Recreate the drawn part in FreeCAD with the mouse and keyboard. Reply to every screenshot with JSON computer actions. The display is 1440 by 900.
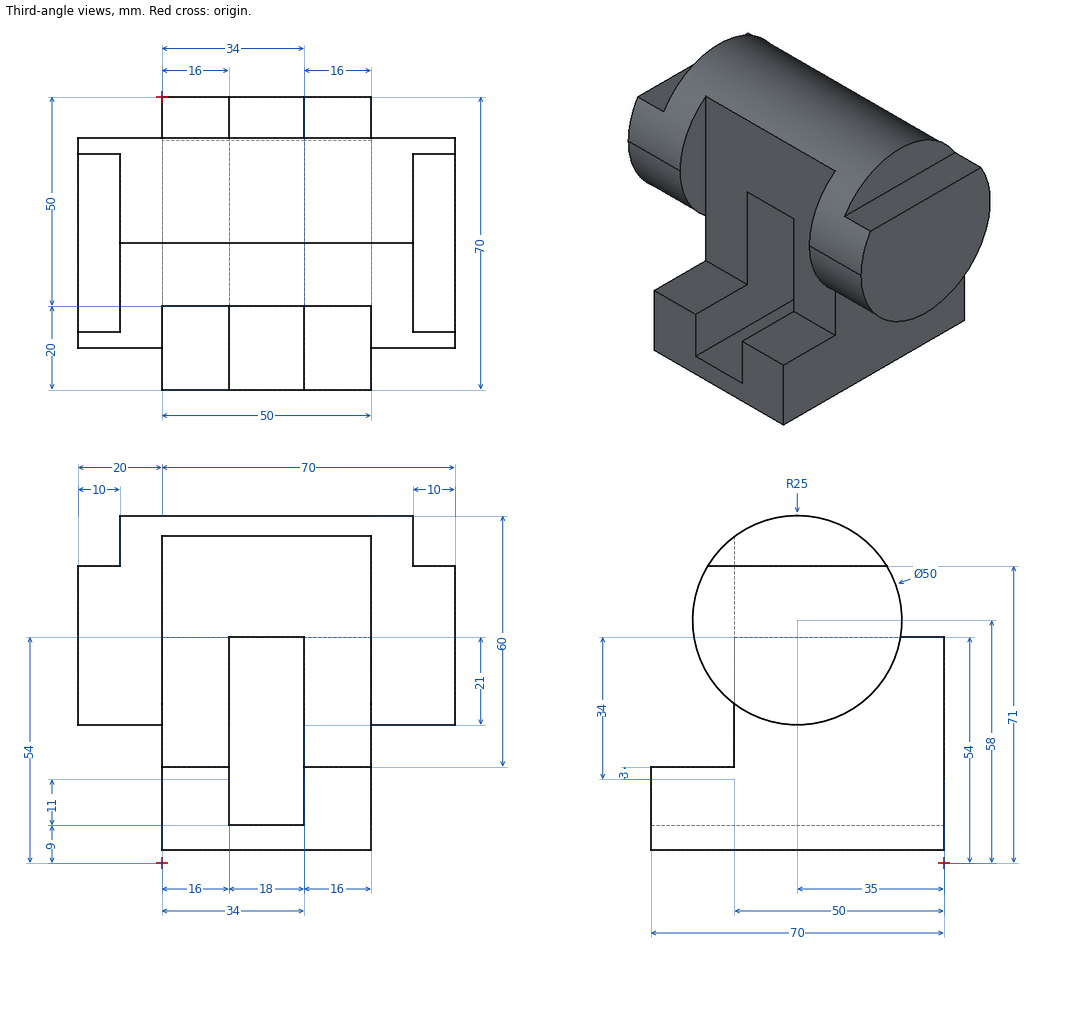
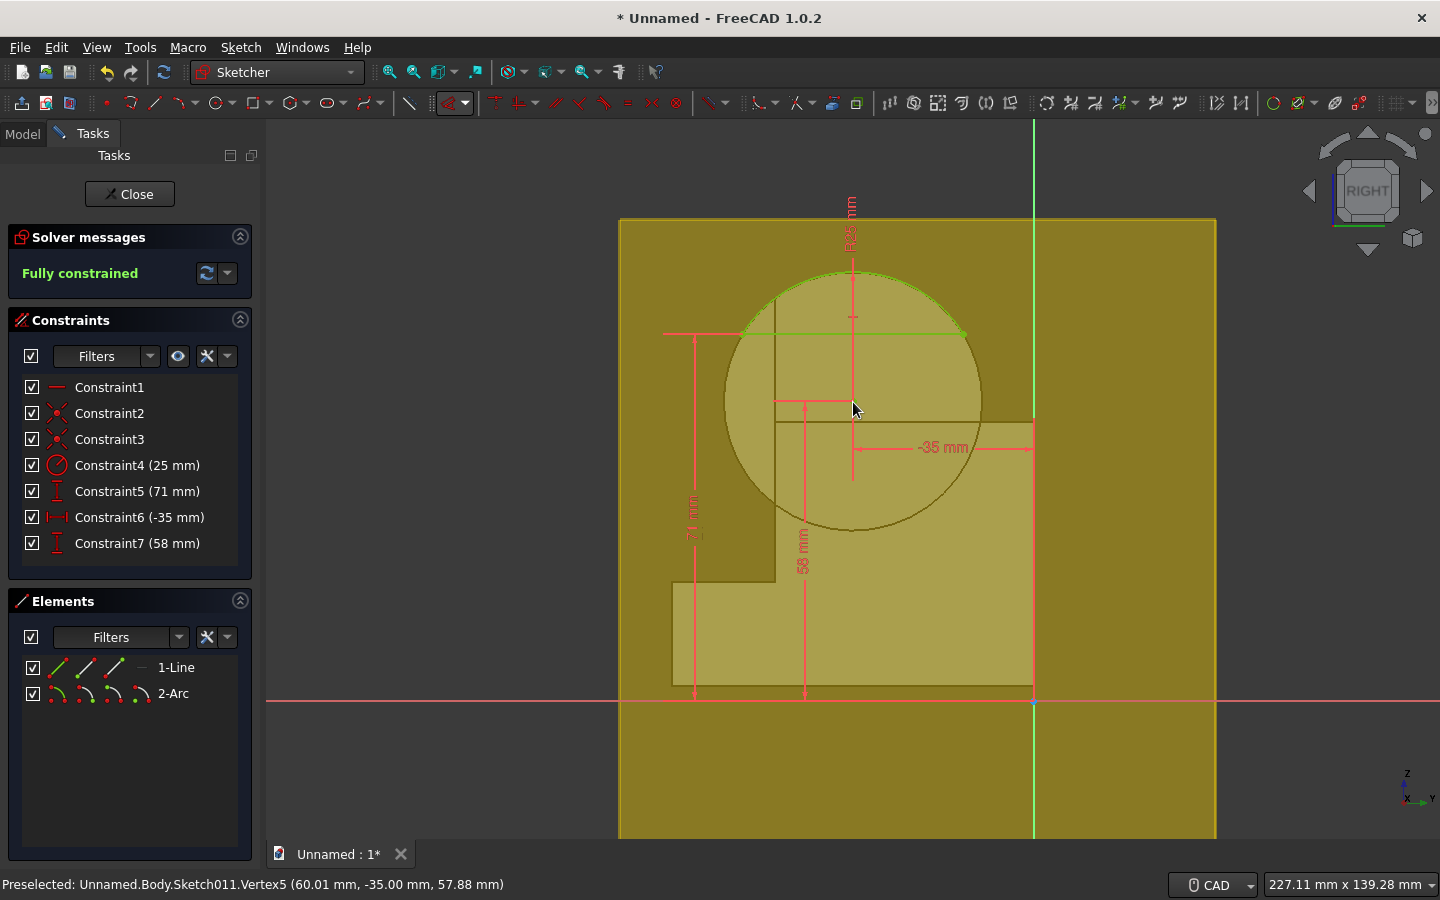
{"action": "left_click", "coordinate": [130, 194]}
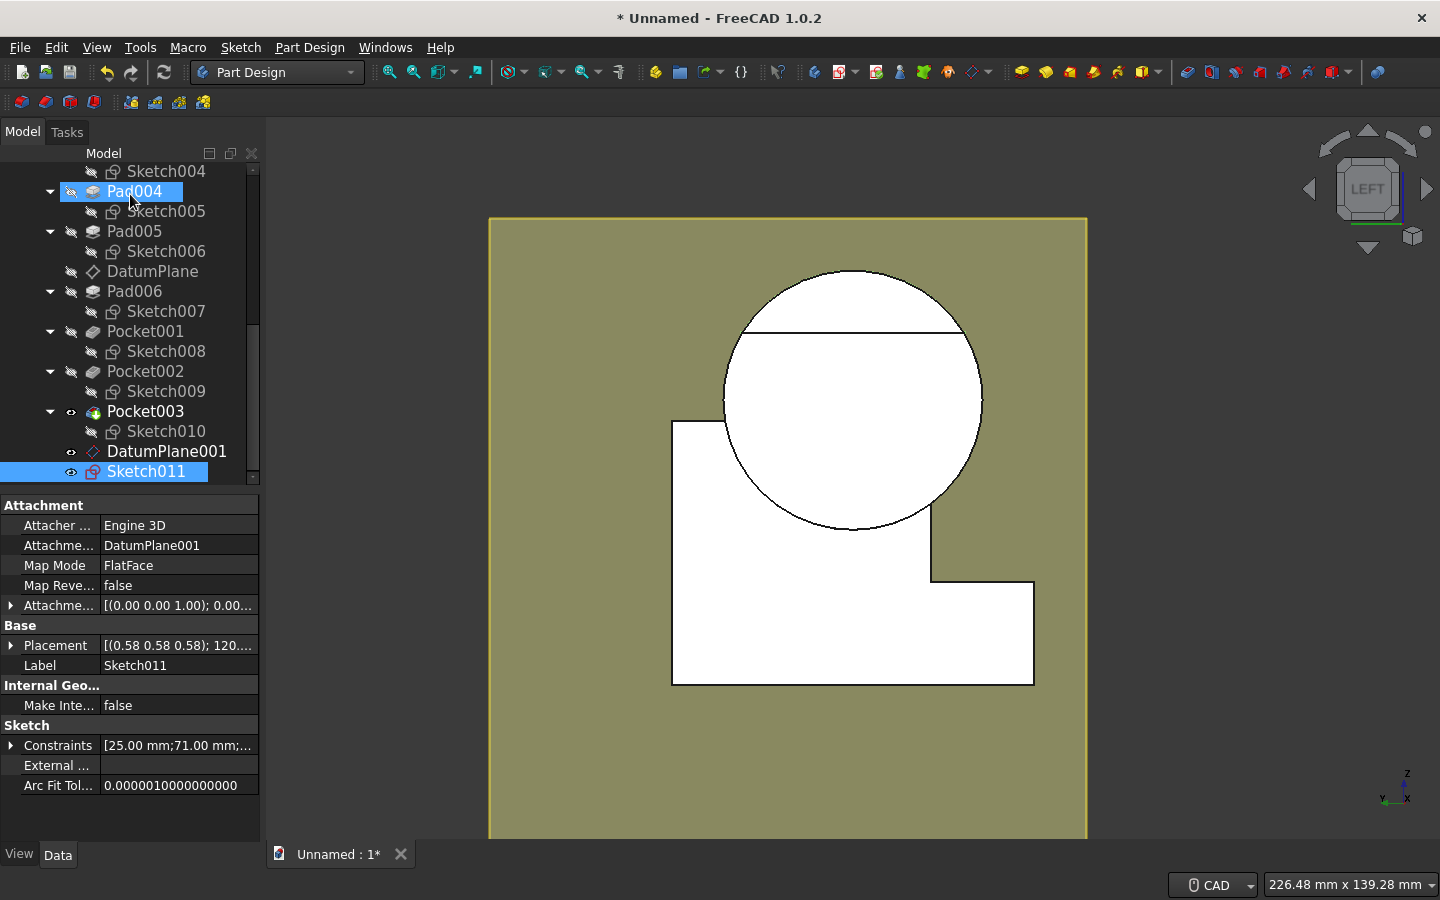
{"action": "left_click", "coordinate": [1188, 72]}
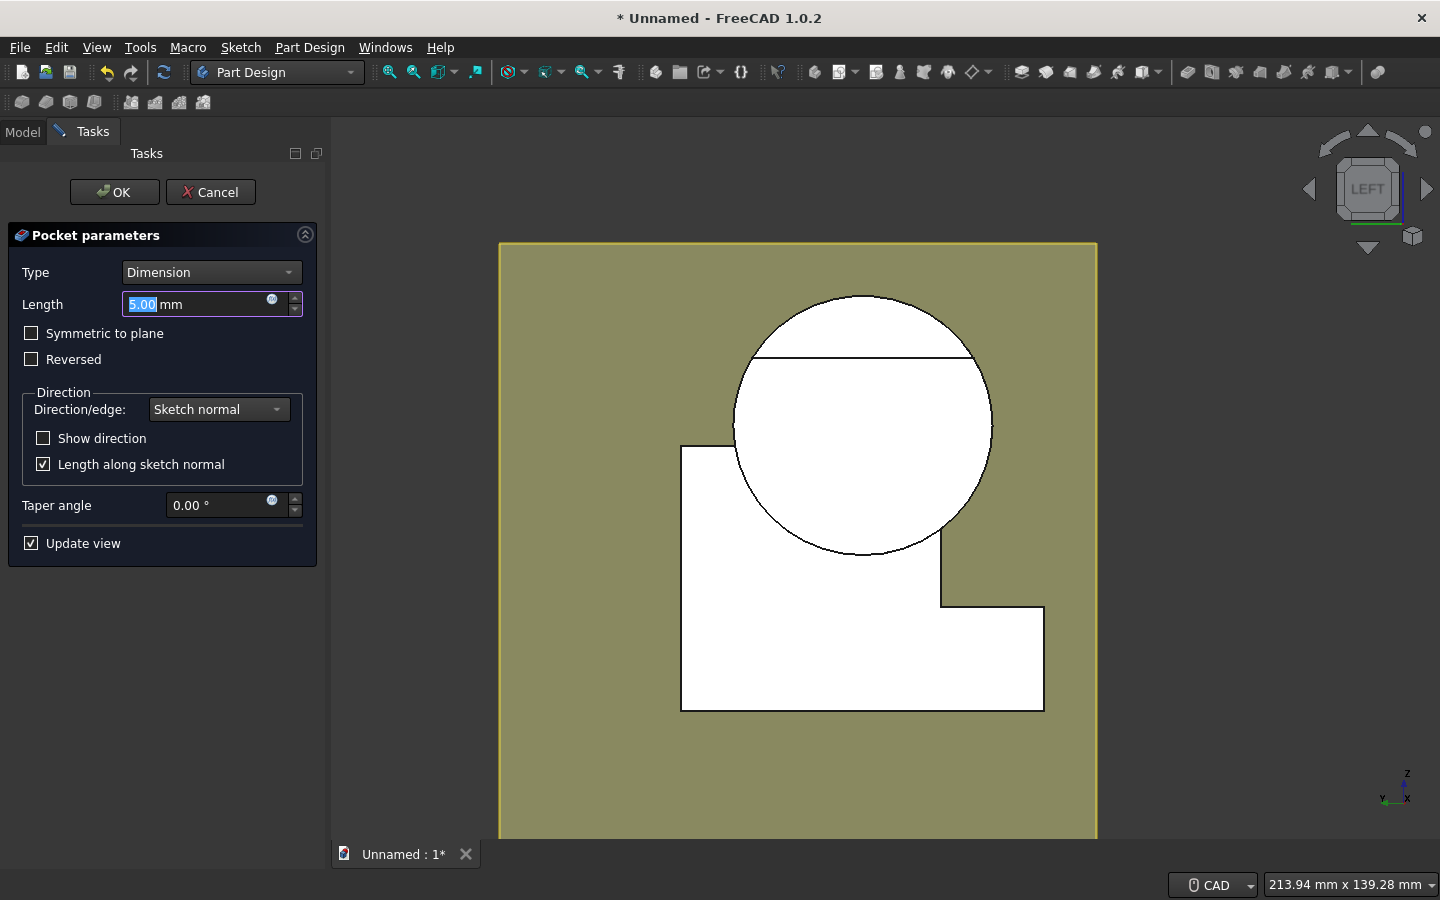
{"action": "type", "text": "10"}
{"action": "key", "text": "Tab"}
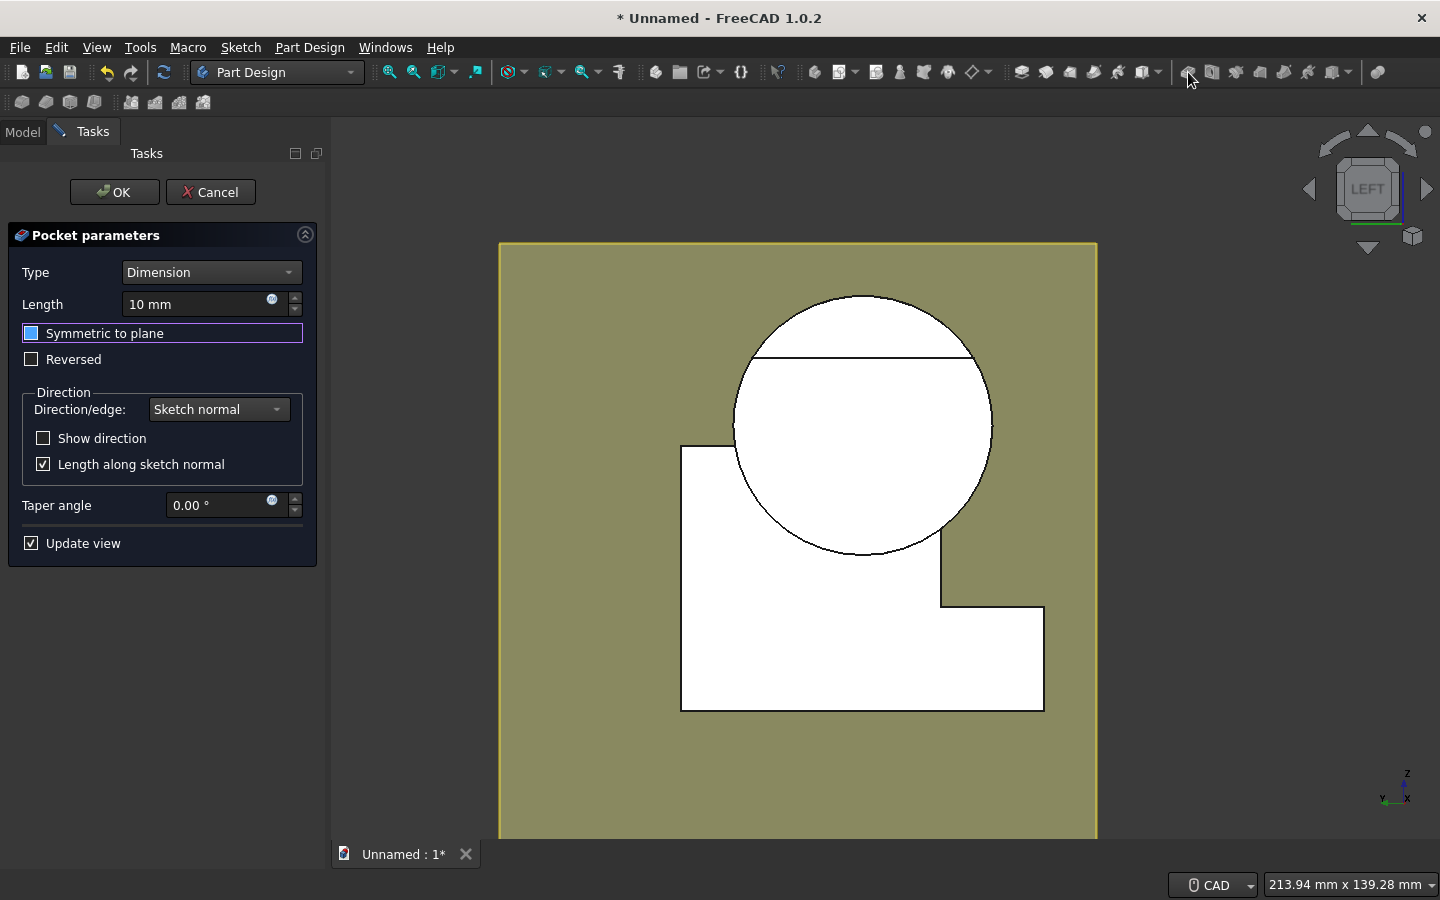
{"action": "left_click", "coordinate": [30, 359]}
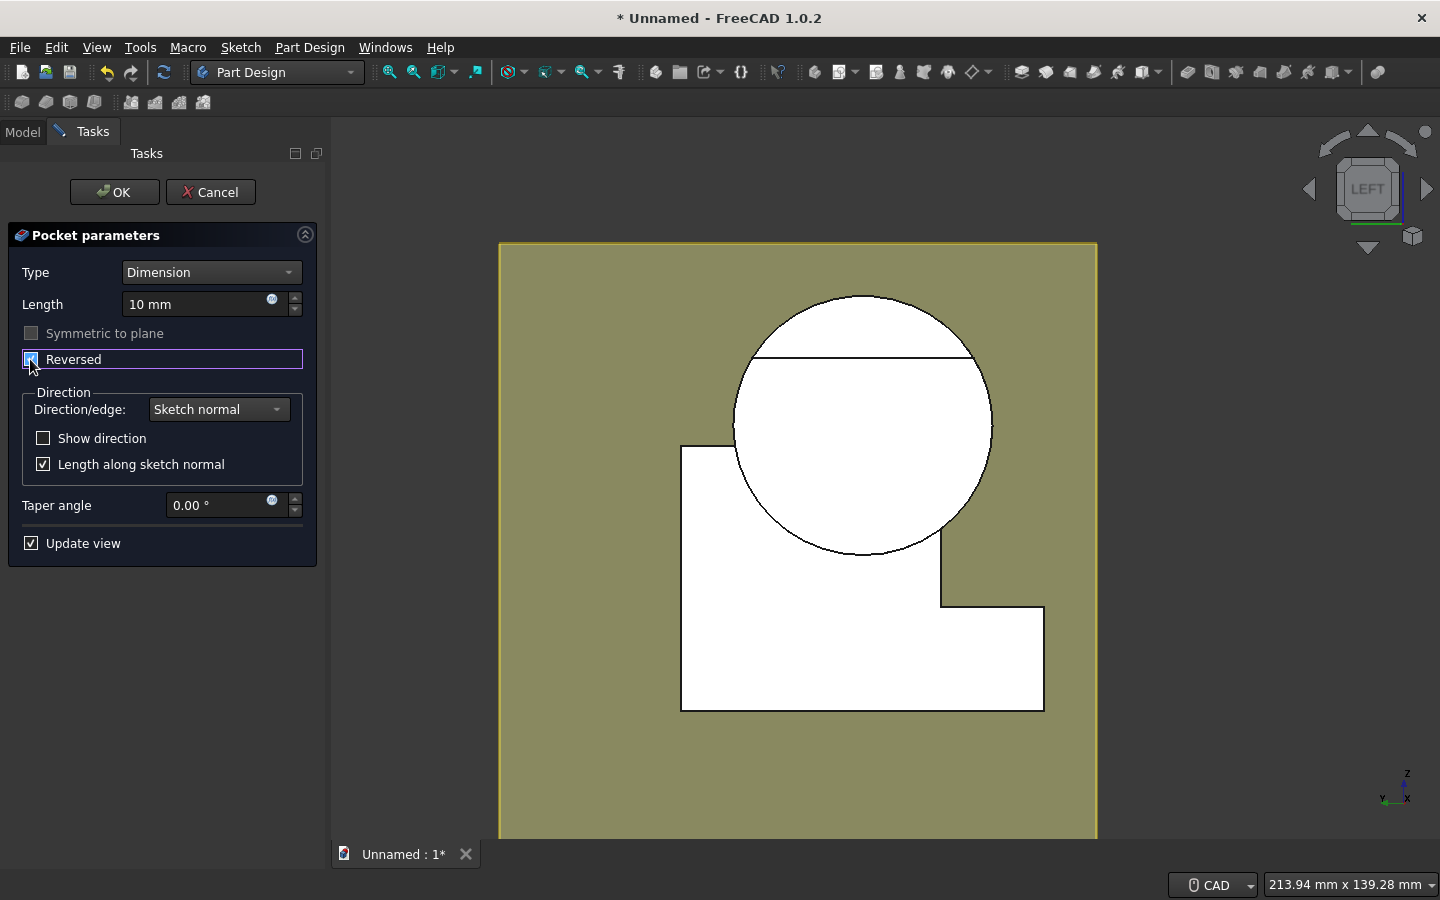
{"action": "left_click", "coordinate": [115, 192]}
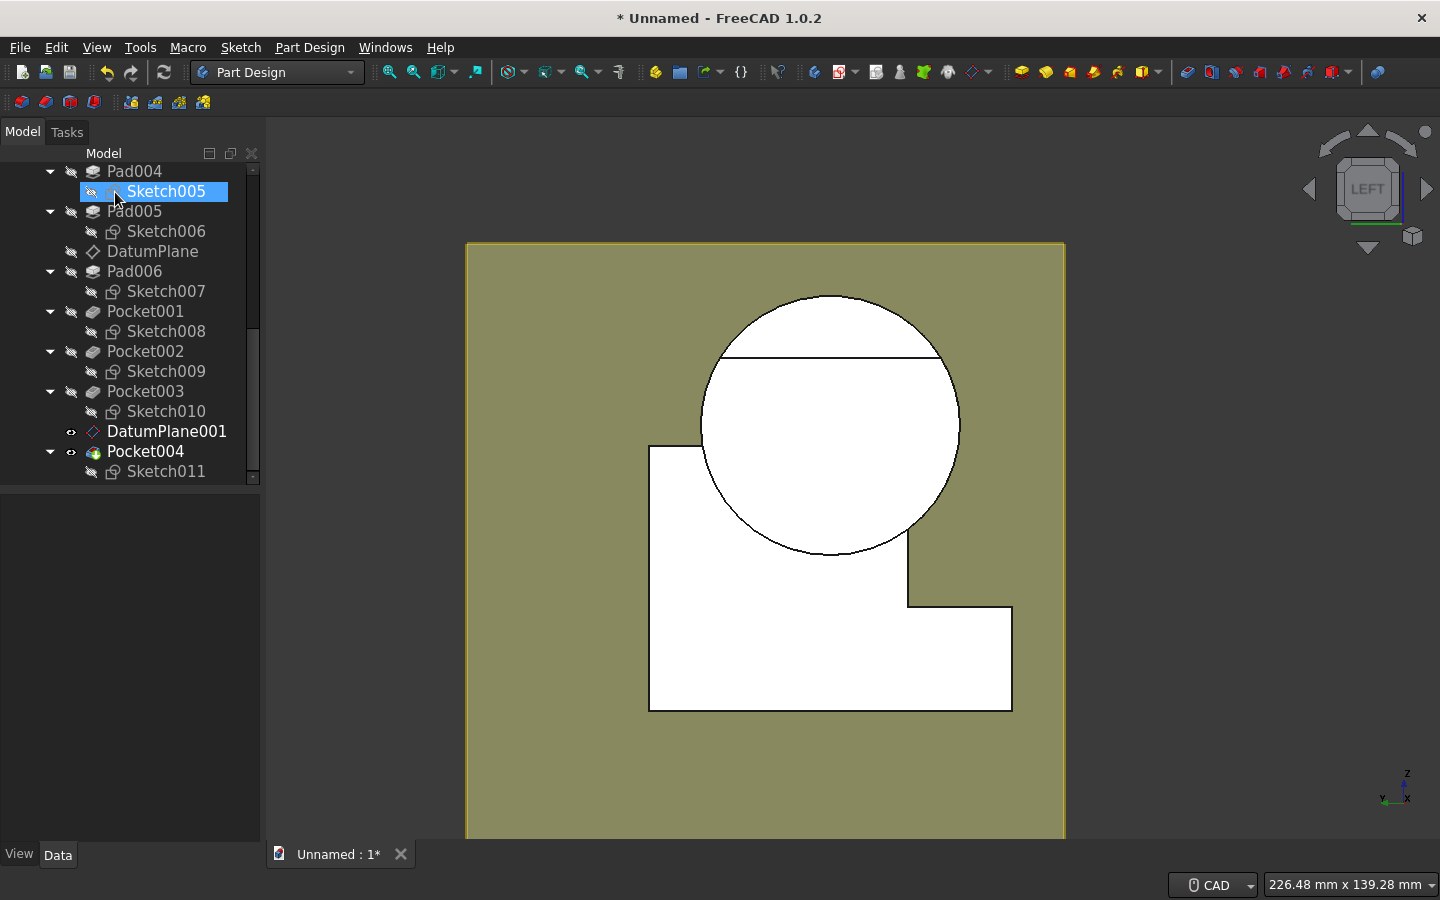
{"action": "left_click", "coordinate": [116, 432]}
{"action": "key", "text": "space"}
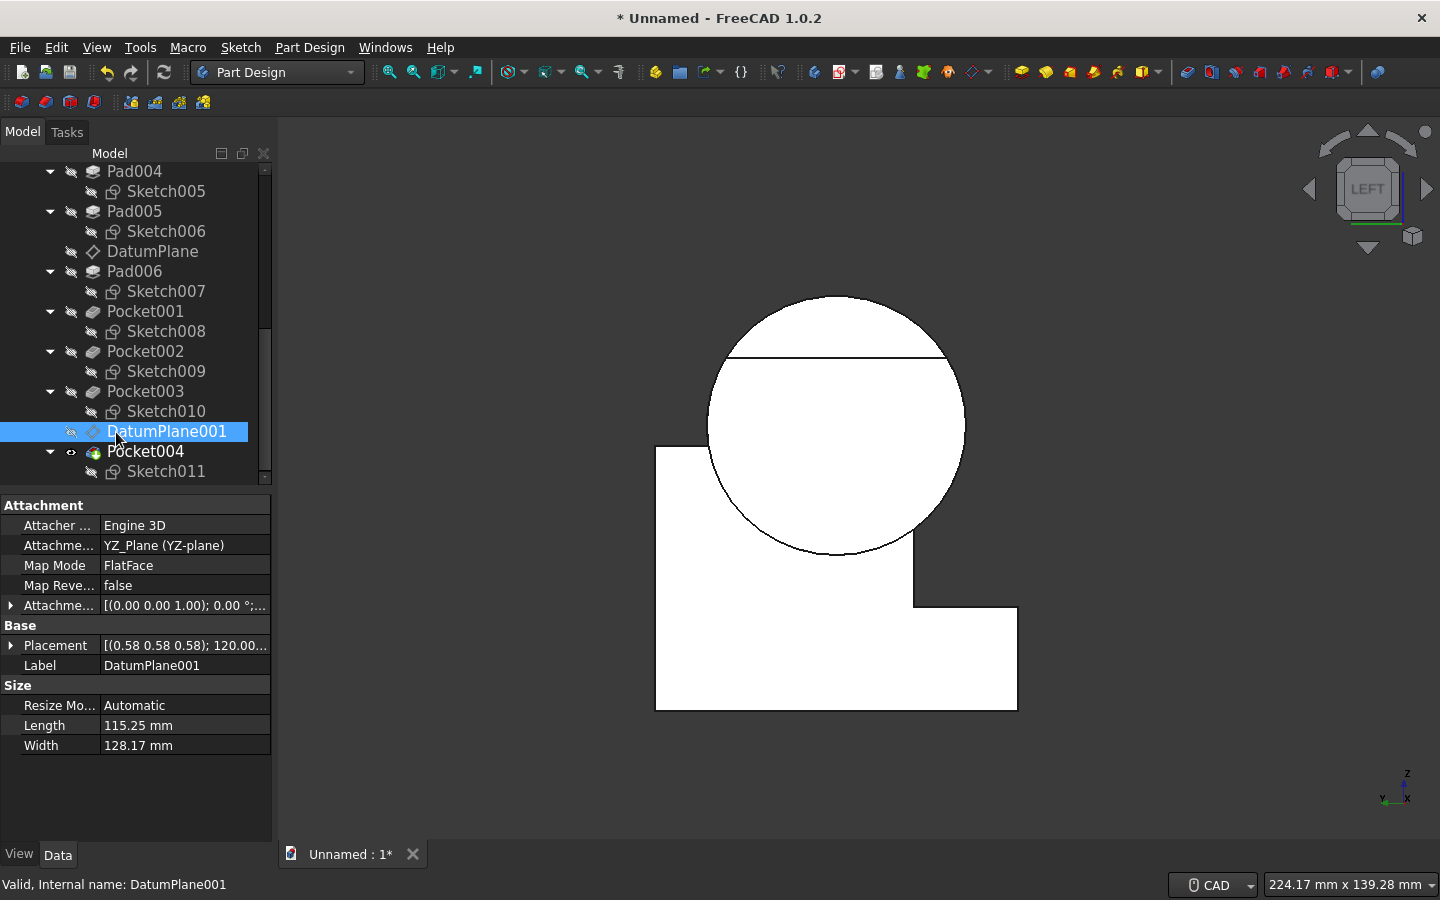
{"action": "key", "text": "0"}